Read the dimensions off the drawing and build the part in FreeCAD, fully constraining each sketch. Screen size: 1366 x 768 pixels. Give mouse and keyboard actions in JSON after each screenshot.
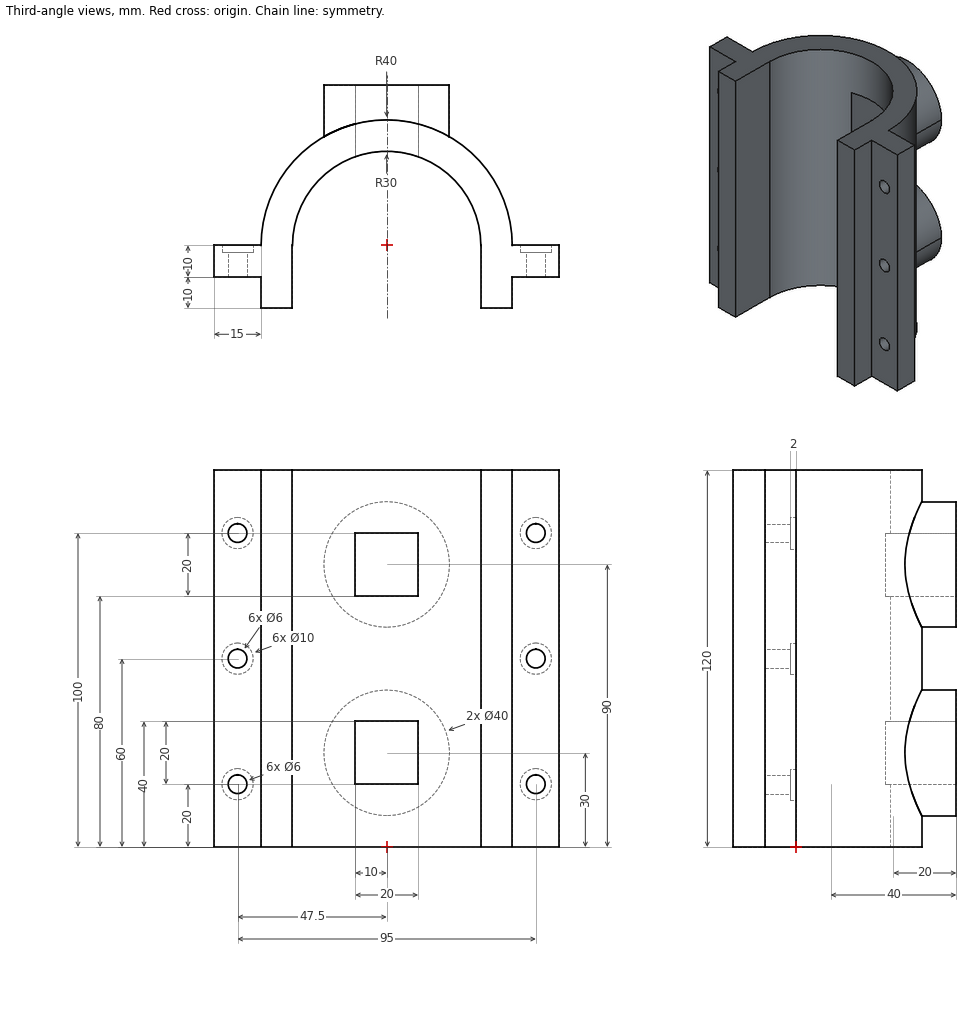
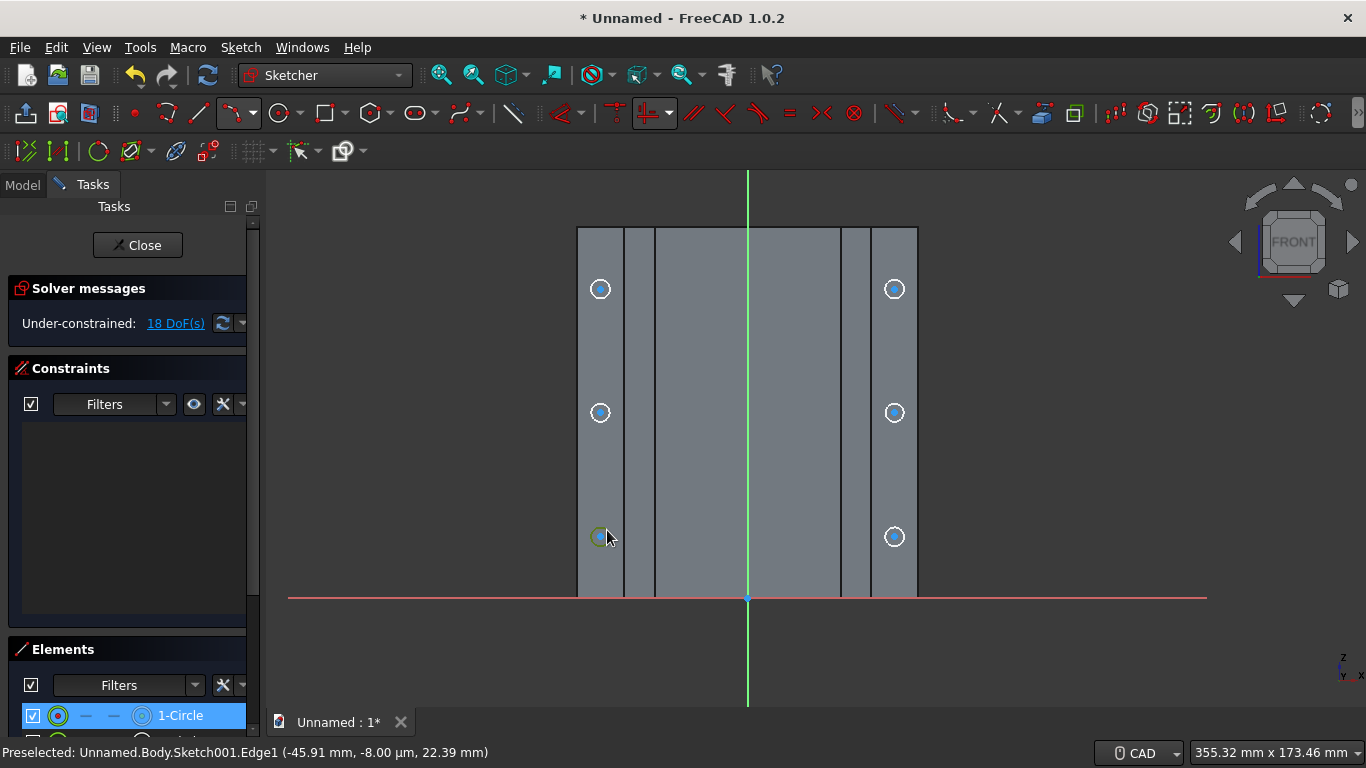
{"action": "scroll", "coordinate": [607, 282], "scroll_direction": "up", "scroll_amount": 2}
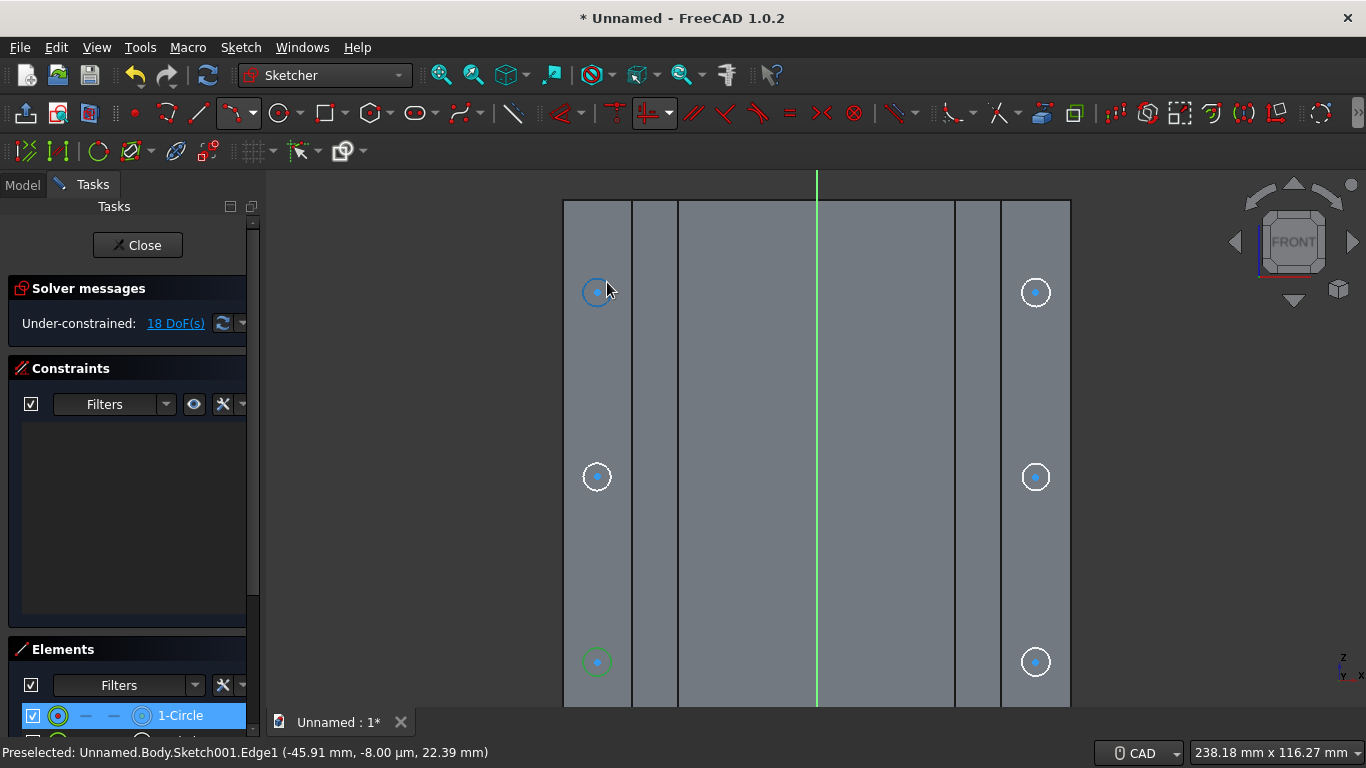
{"action": "left_click", "coordinate": [607, 283]}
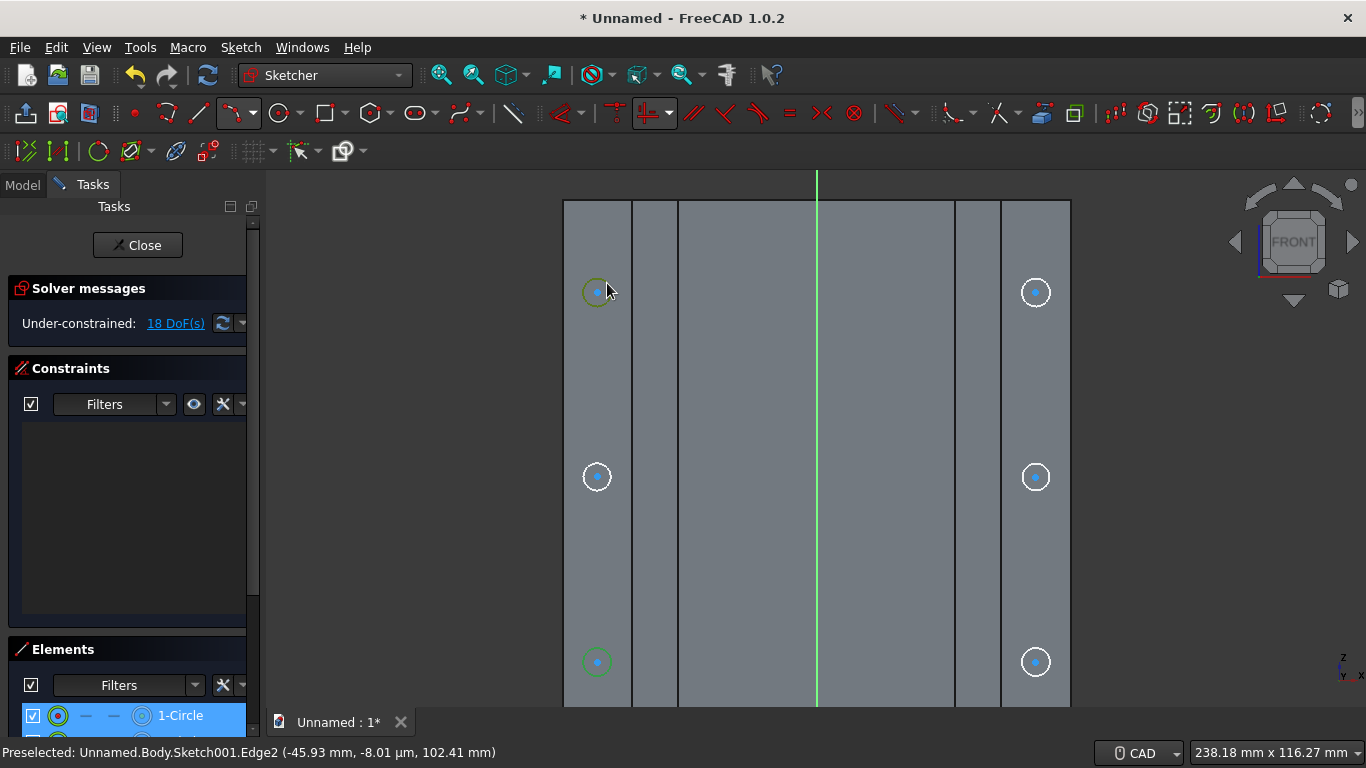
{"action": "left_click", "coordinate": [607, 467]}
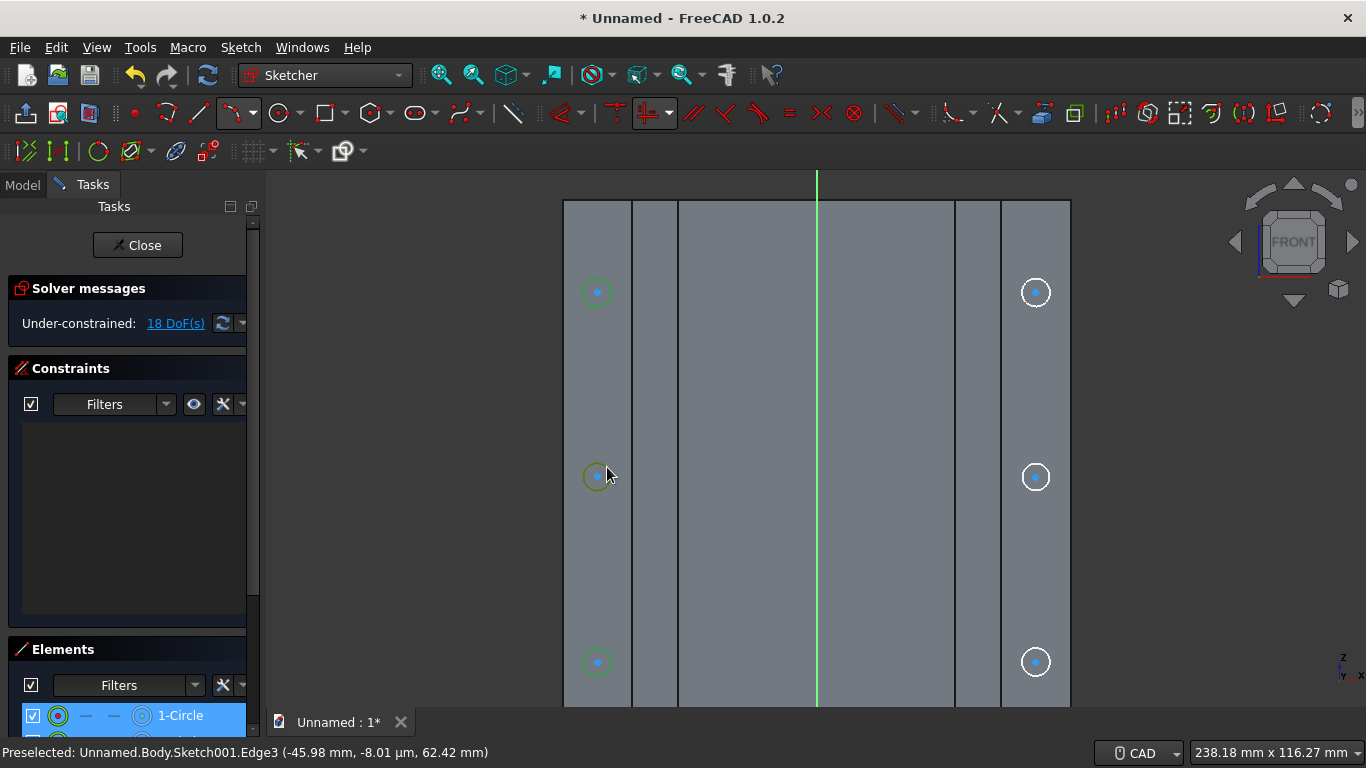
{"action": "left_click", "coordinate": [1046, 652]}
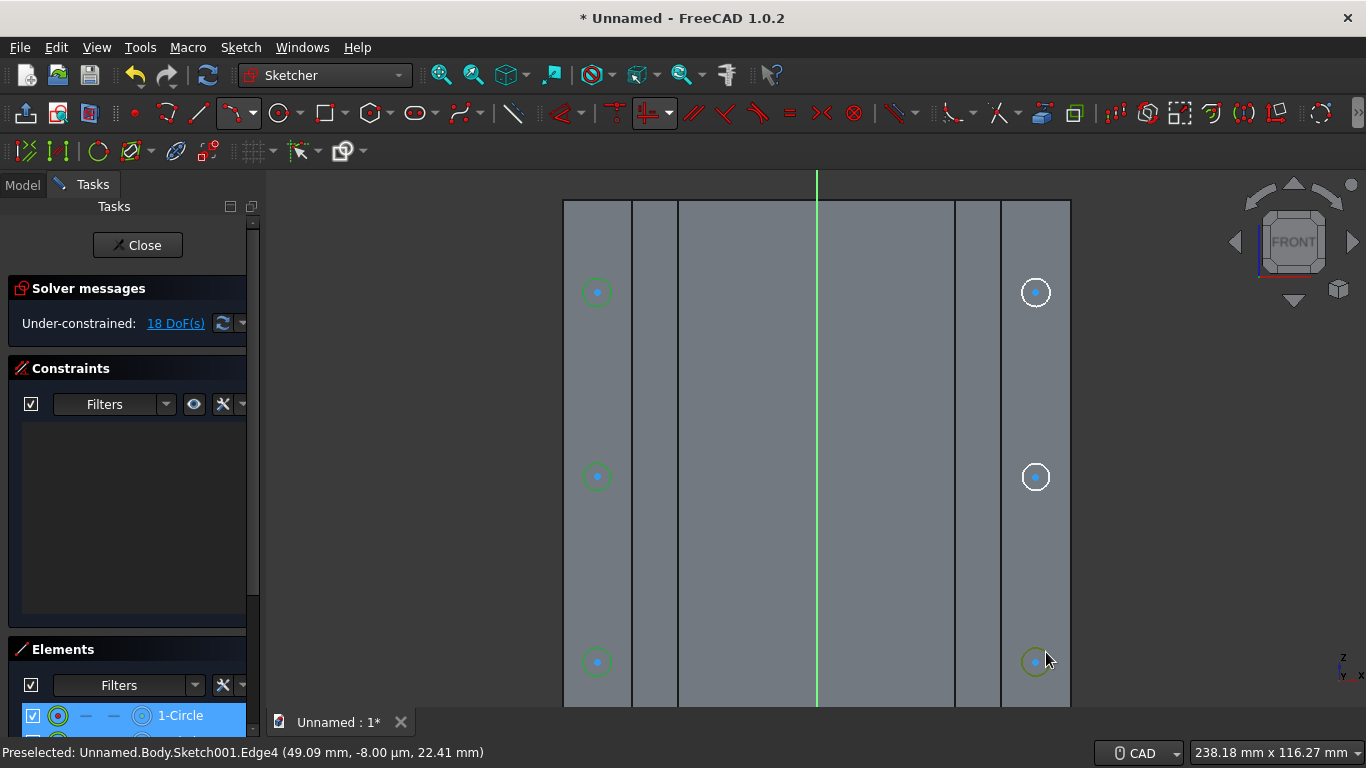
{"action": "left_click", "coordinate": [1045, 468]}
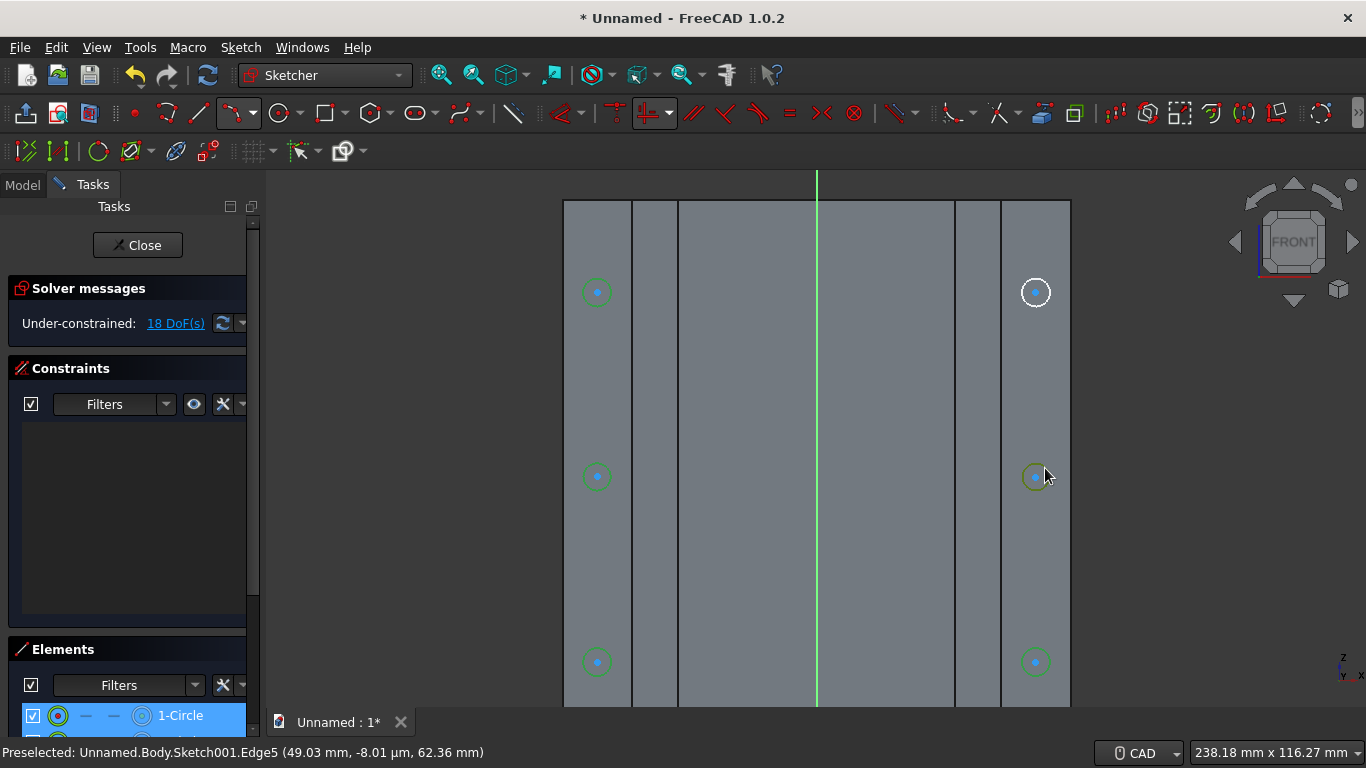
{"action": "left_click", "coordinate": [1046, 283]}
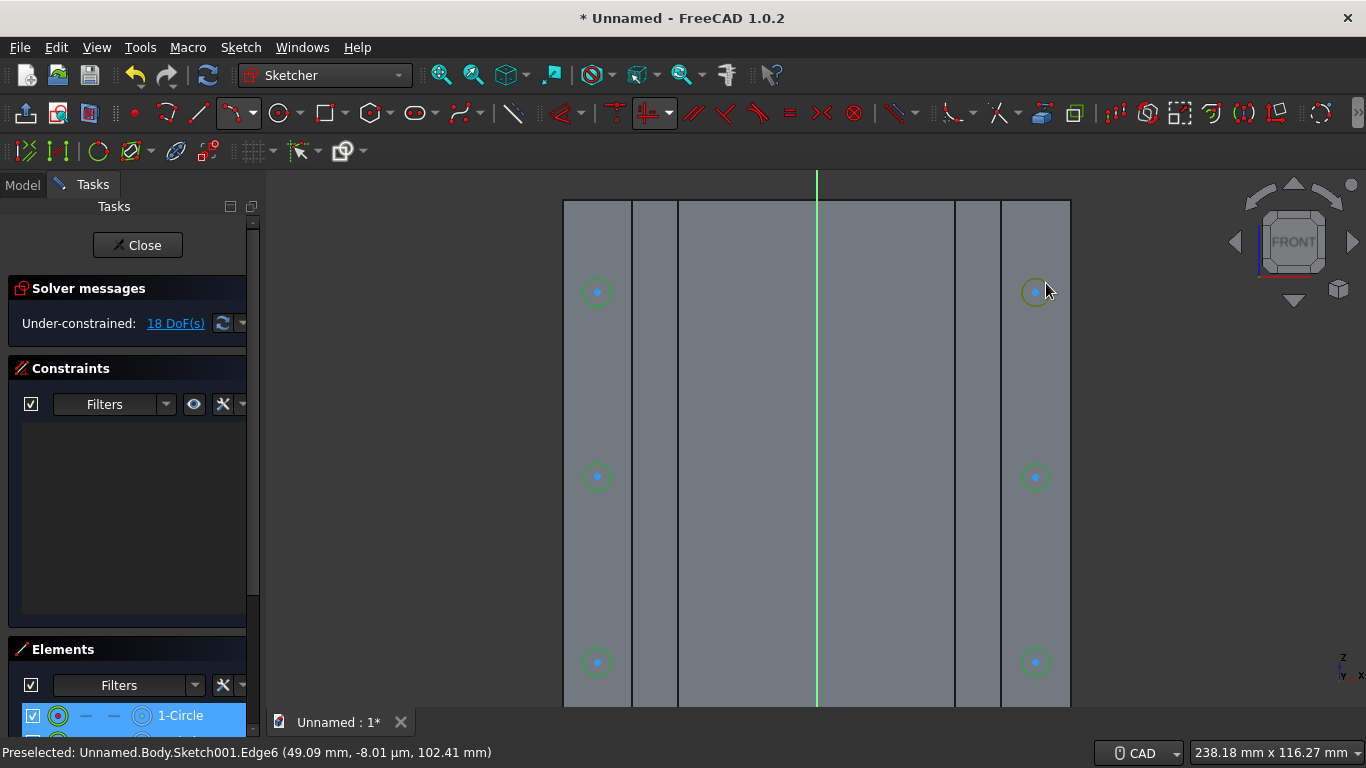
{"action": "left_click", "coordinate": [790, 114]}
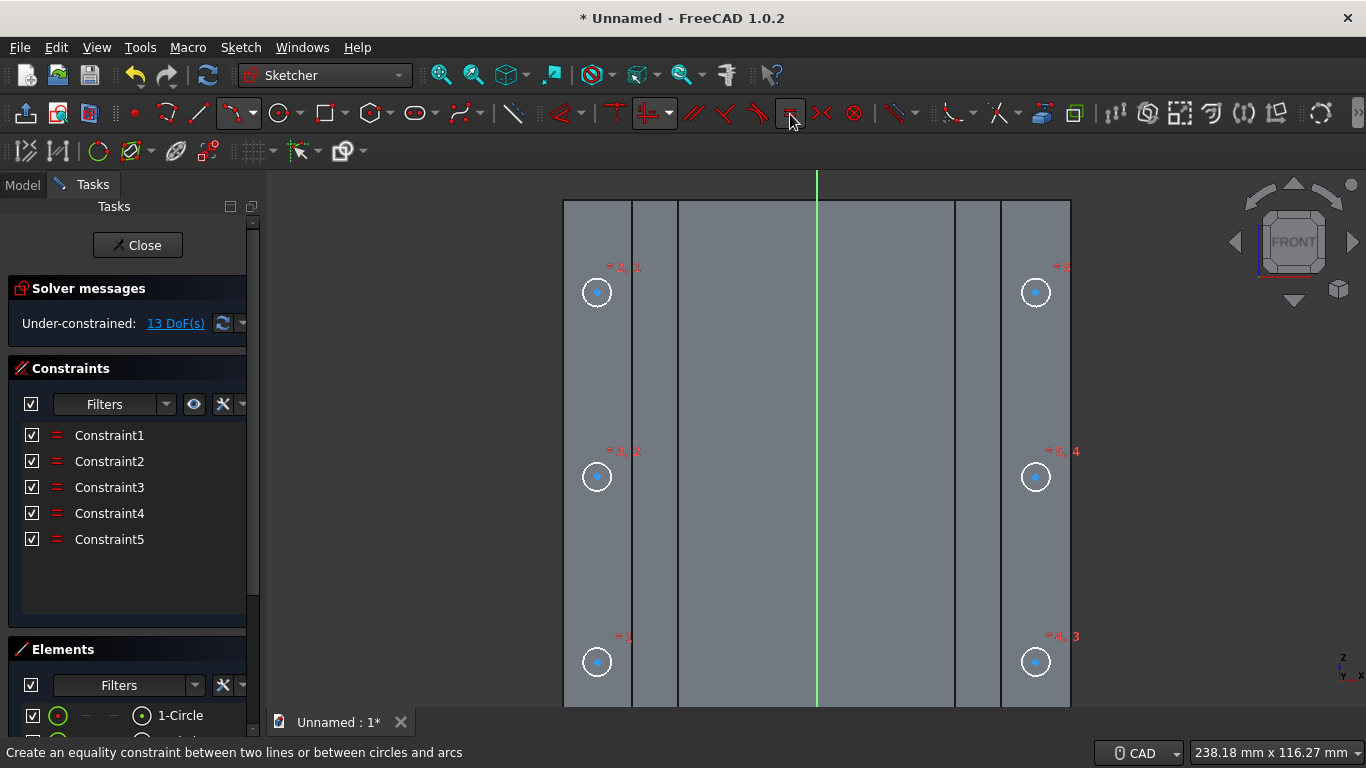
{"action": "left_click", "coordinate": [597, 662]}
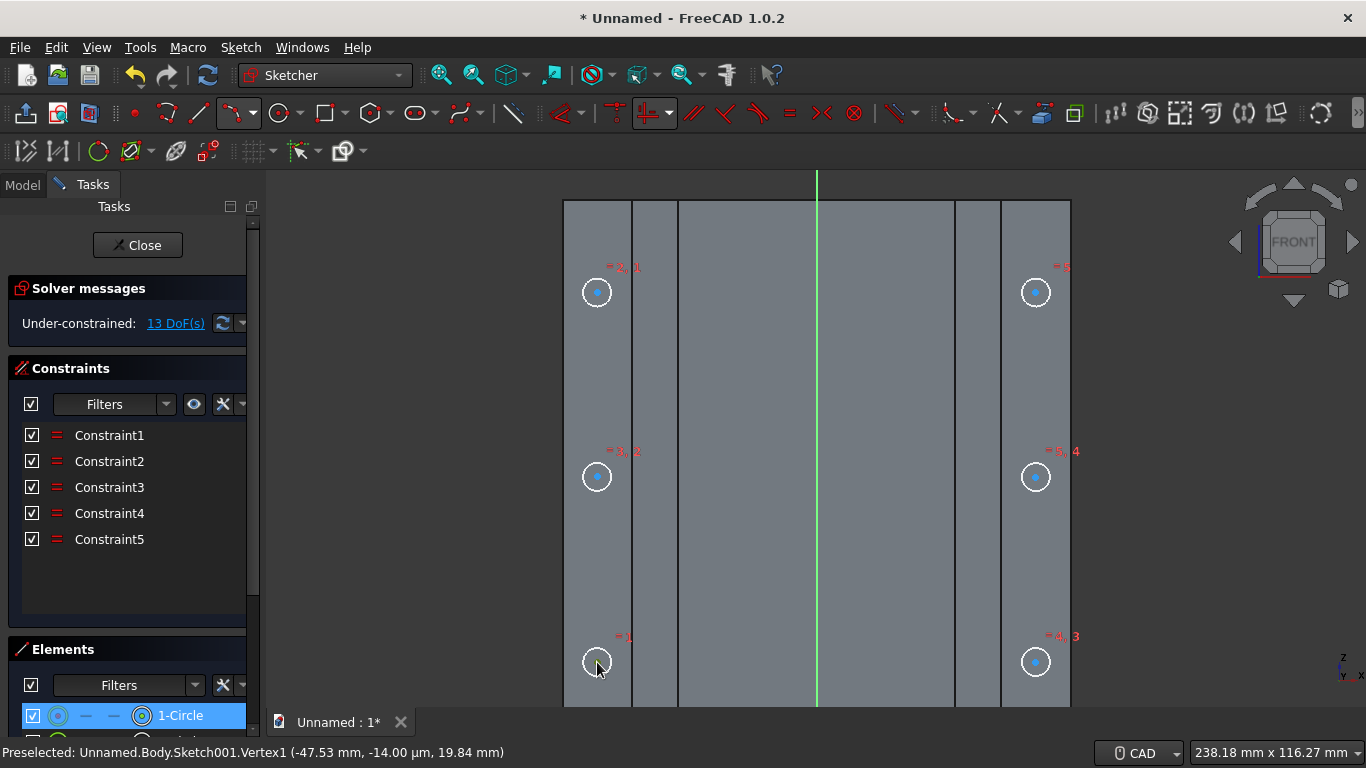
{"action": "left_click", "coordinate": [597, 293]}